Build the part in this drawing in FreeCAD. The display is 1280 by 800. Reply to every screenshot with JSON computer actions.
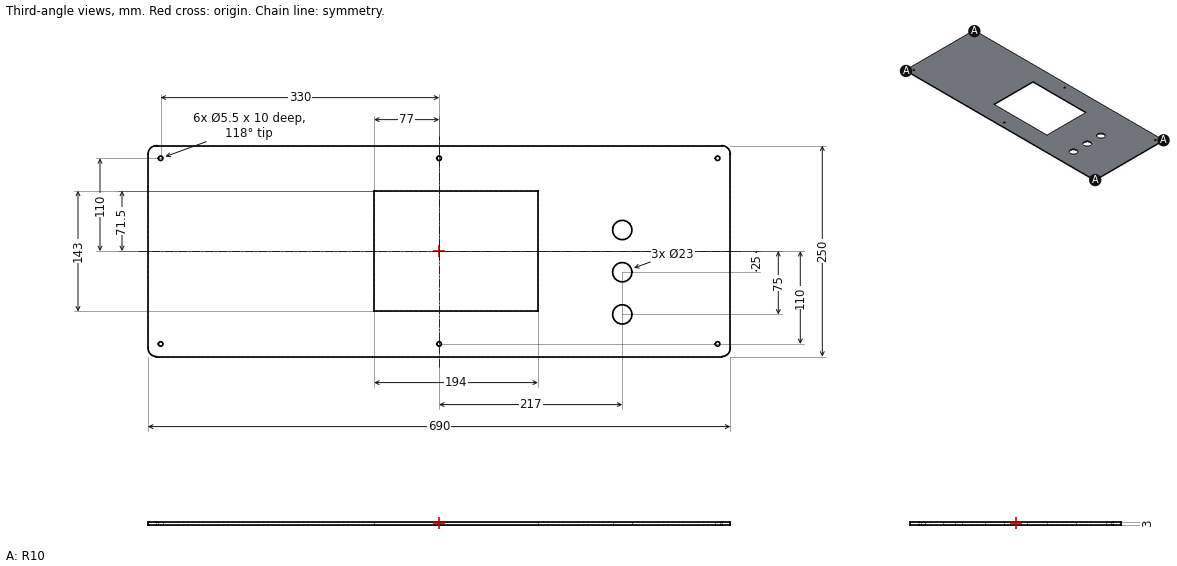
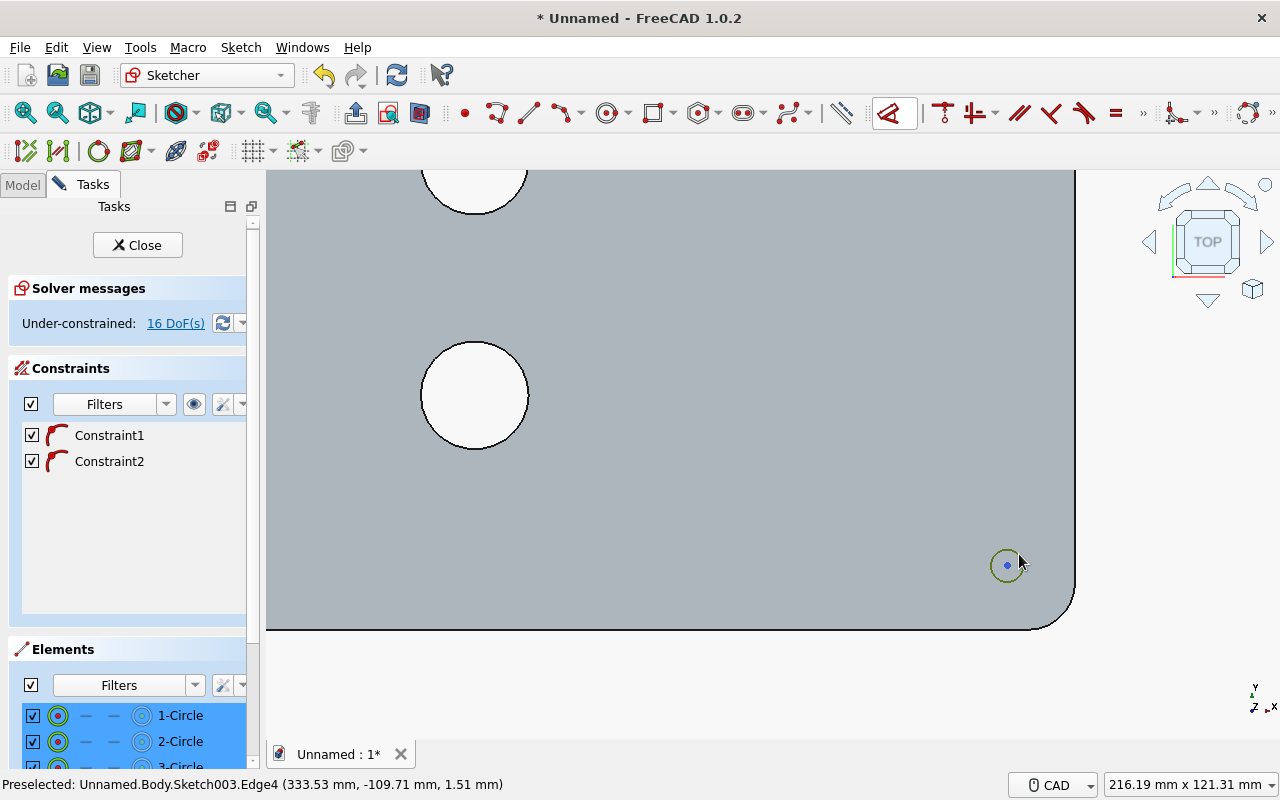
{"action": "scroll", "coordinate": [1020, 558], "scroll_direction": "down", "scroll_amount": 8}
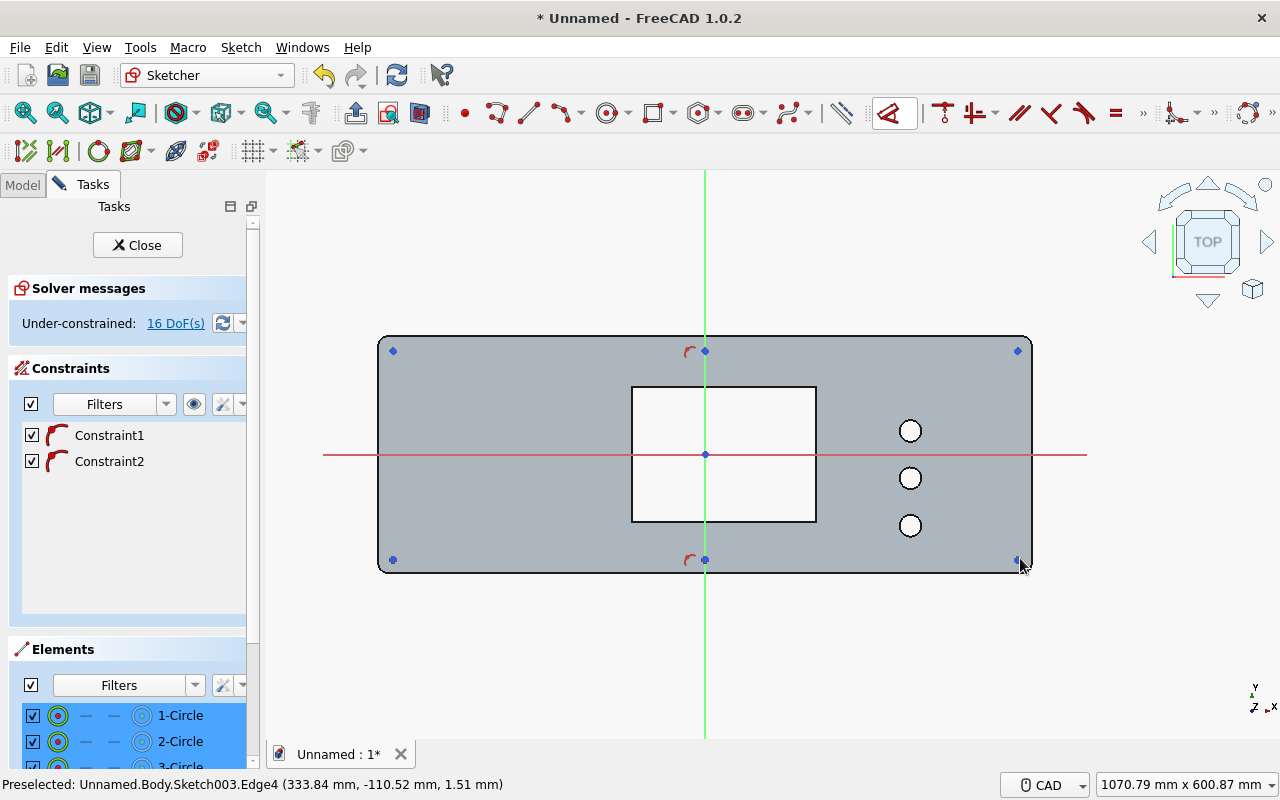
{"action": "scroll", "coordinate": [707, 558], "scroll_direction": "up", "scroll_amount": 10}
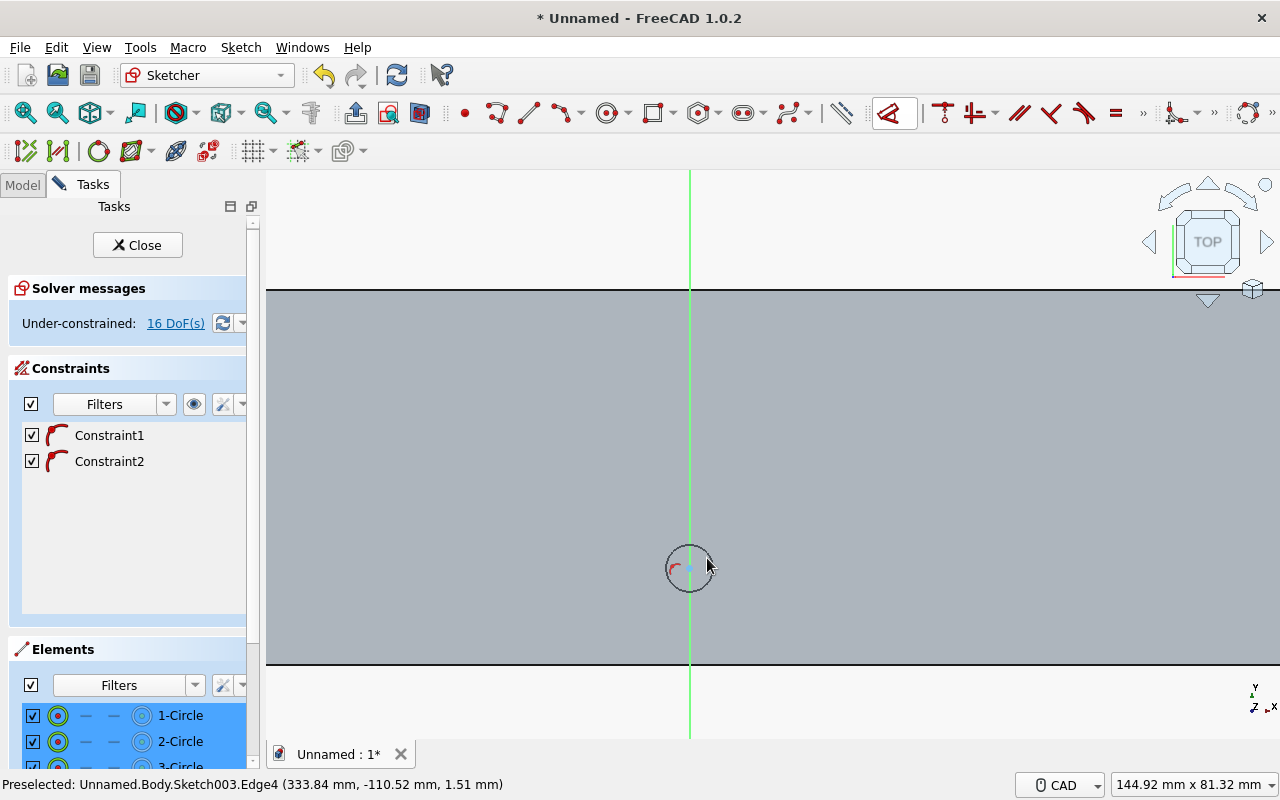
{"action": "left_click", "coordinate": [706, 552]}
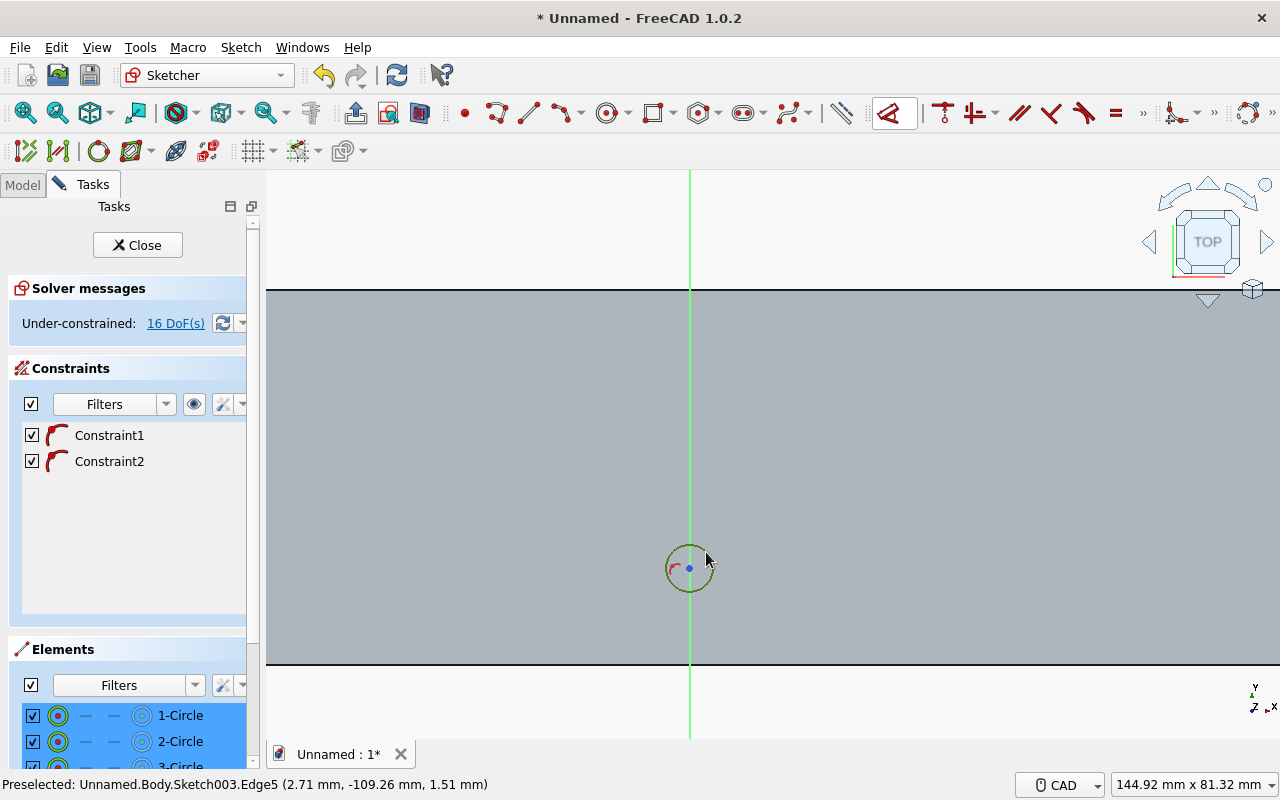
{"action": "scroll", "coordinate": [707, 558], "scroll_direction": "down", "scroll_amount": 10}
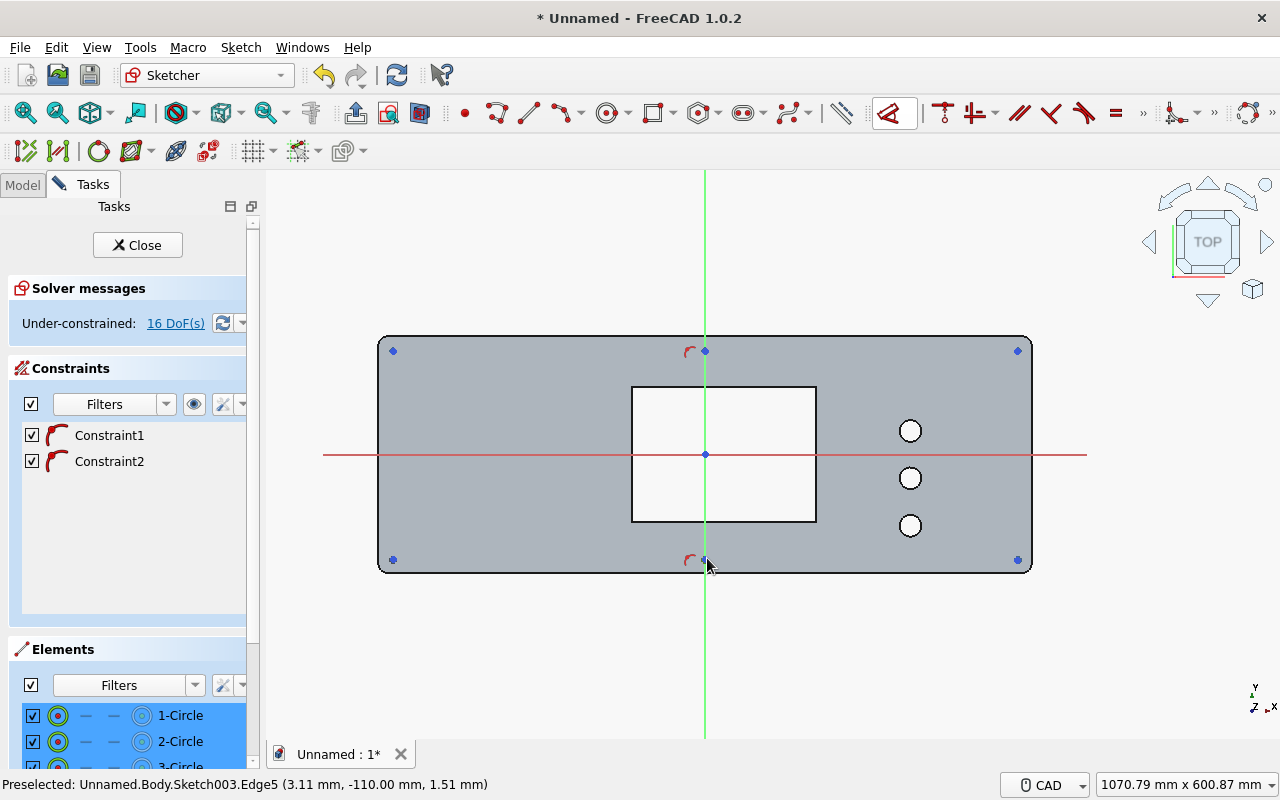
{"action": "scroll", "coordinate": [395, 558], "scroll_direction": "up", "scroll_amount": 8}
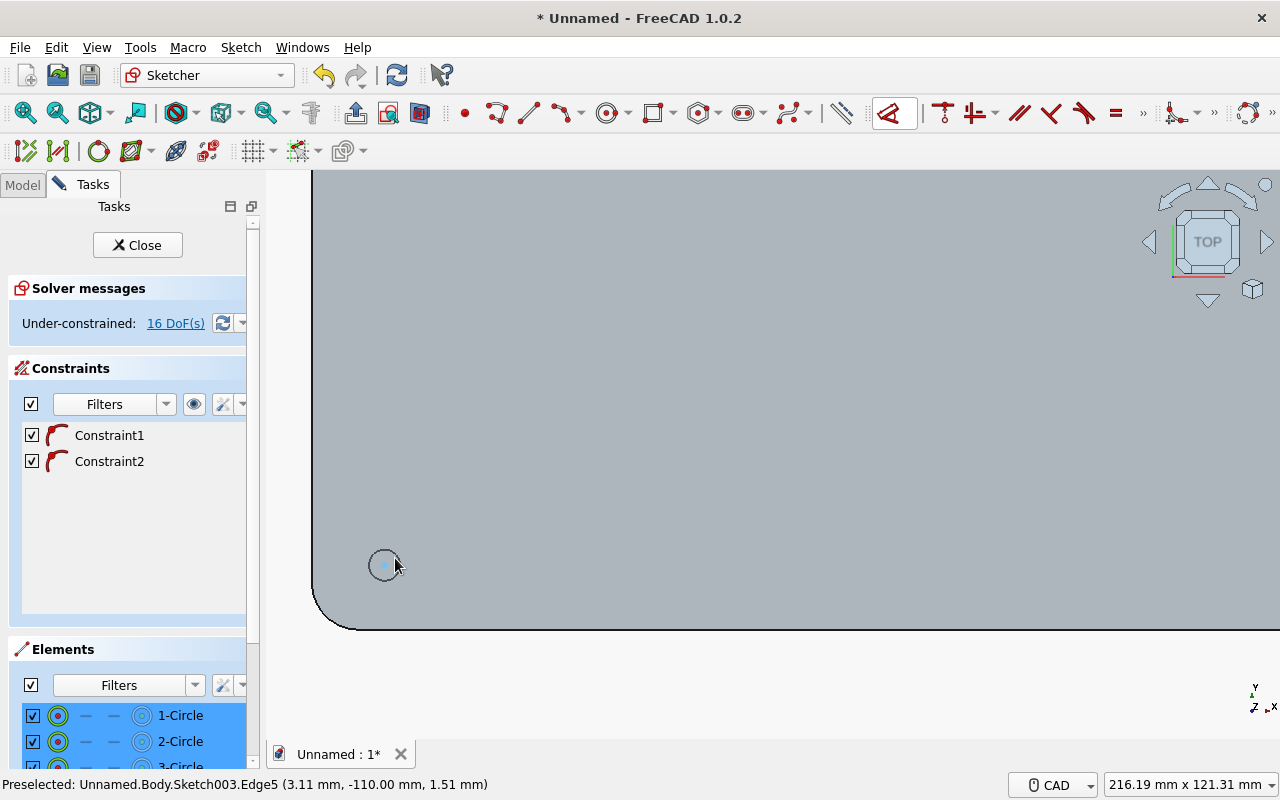
{"action": "left_click", "coordinate": [396, 554]}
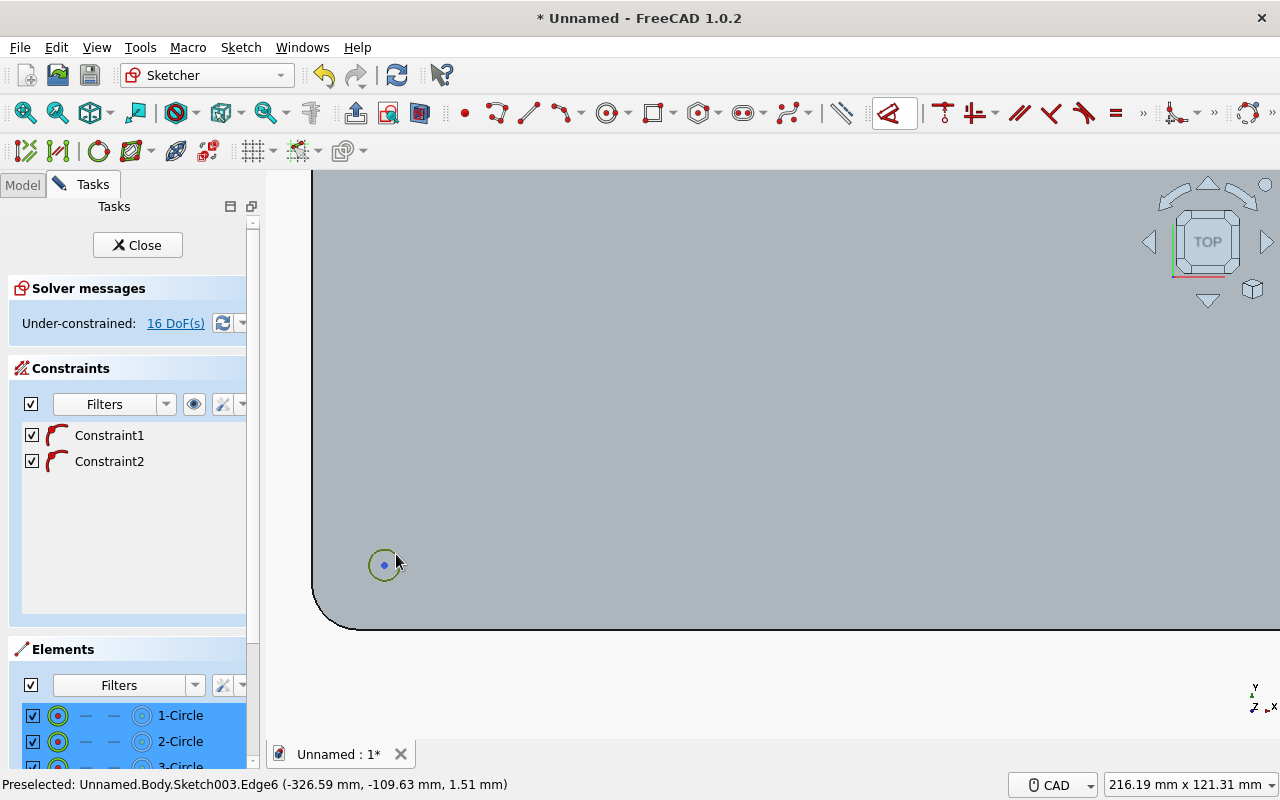
{"action": "left_click", "coordinate": [1116, 114]}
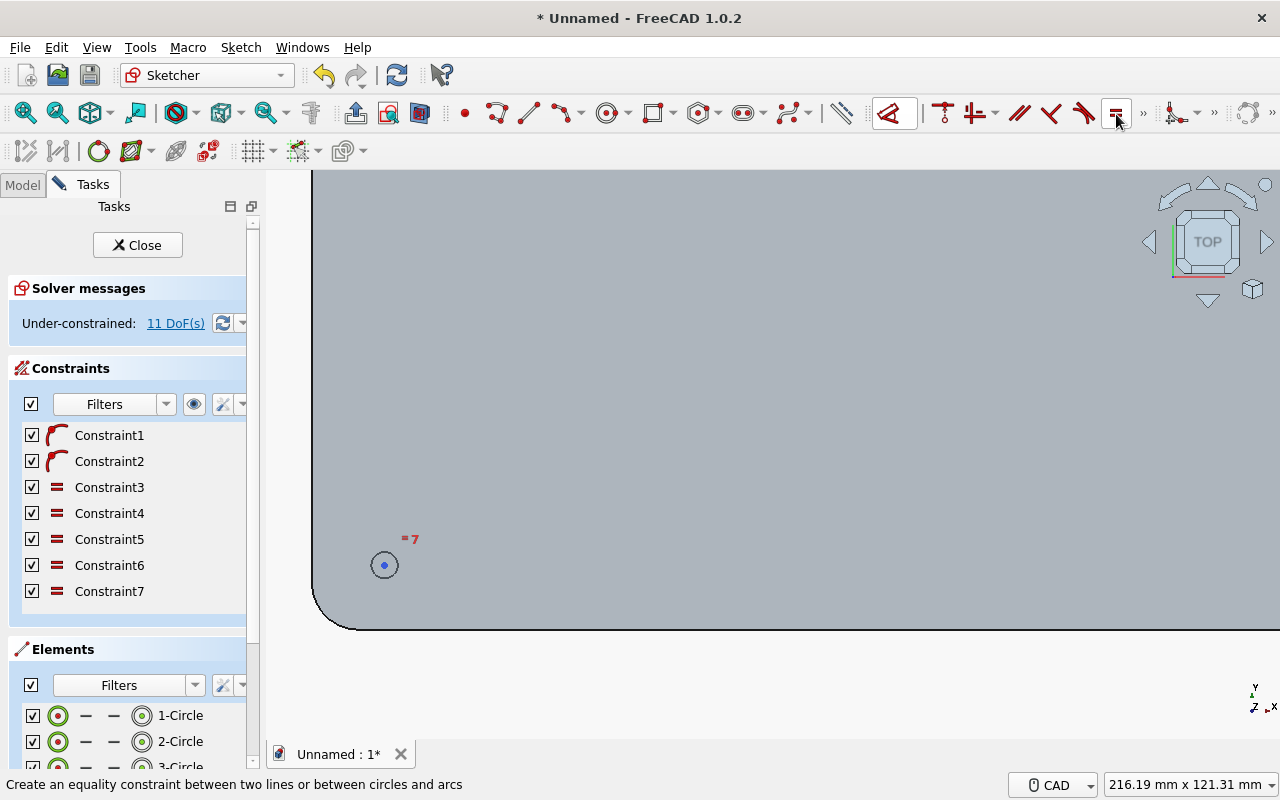
{"action": "scroll", "coordinate": [394, 558], "scroll_direction": "down", "scroll_amount": 8}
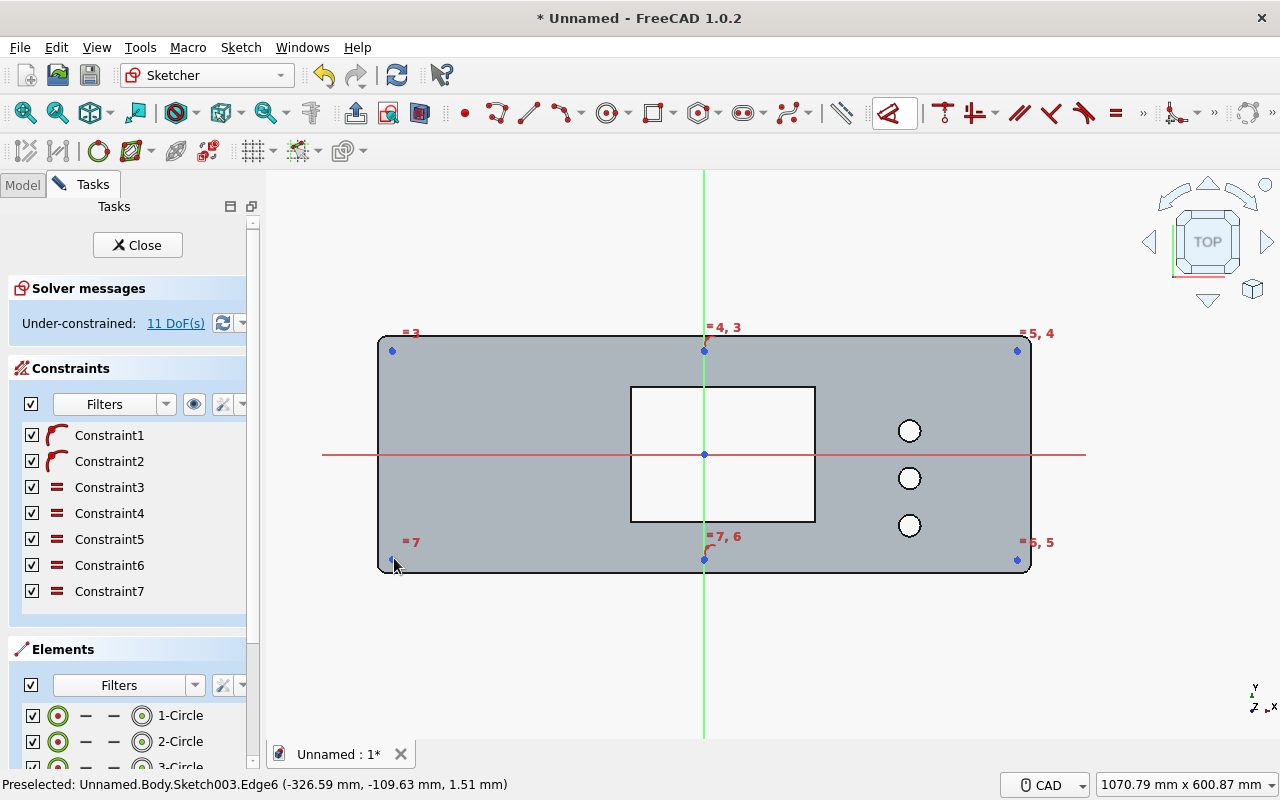
{"action": "left_click", "coordinate": [392, 351]}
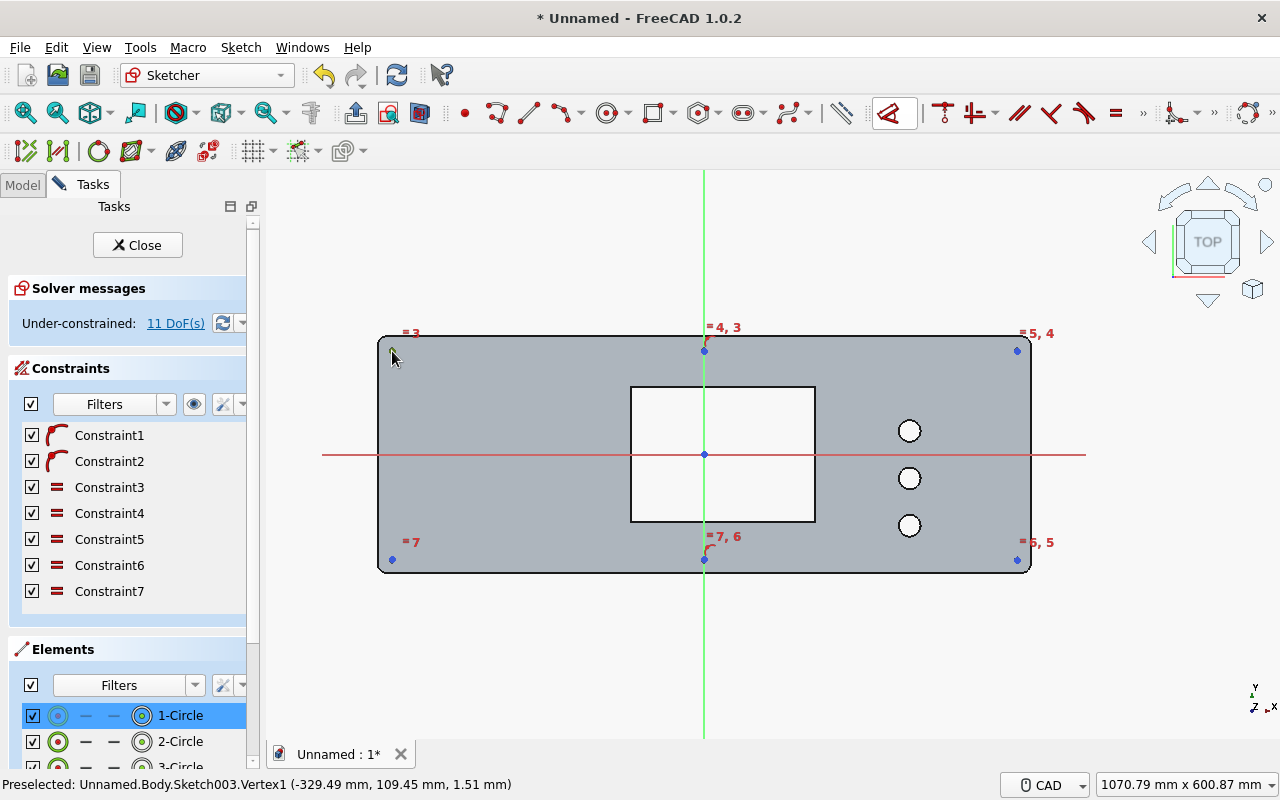
{"action": "left_click", "coordinate": [1017, 351]}